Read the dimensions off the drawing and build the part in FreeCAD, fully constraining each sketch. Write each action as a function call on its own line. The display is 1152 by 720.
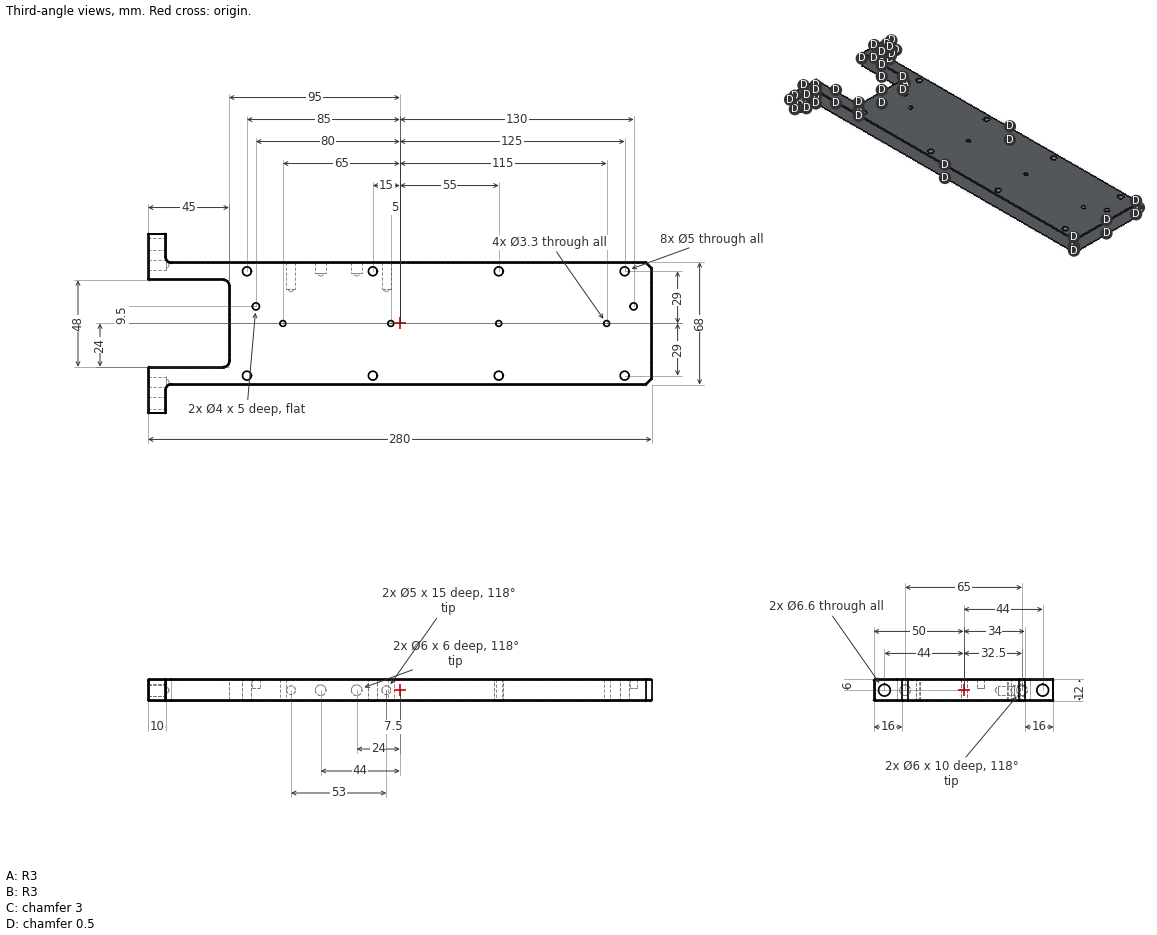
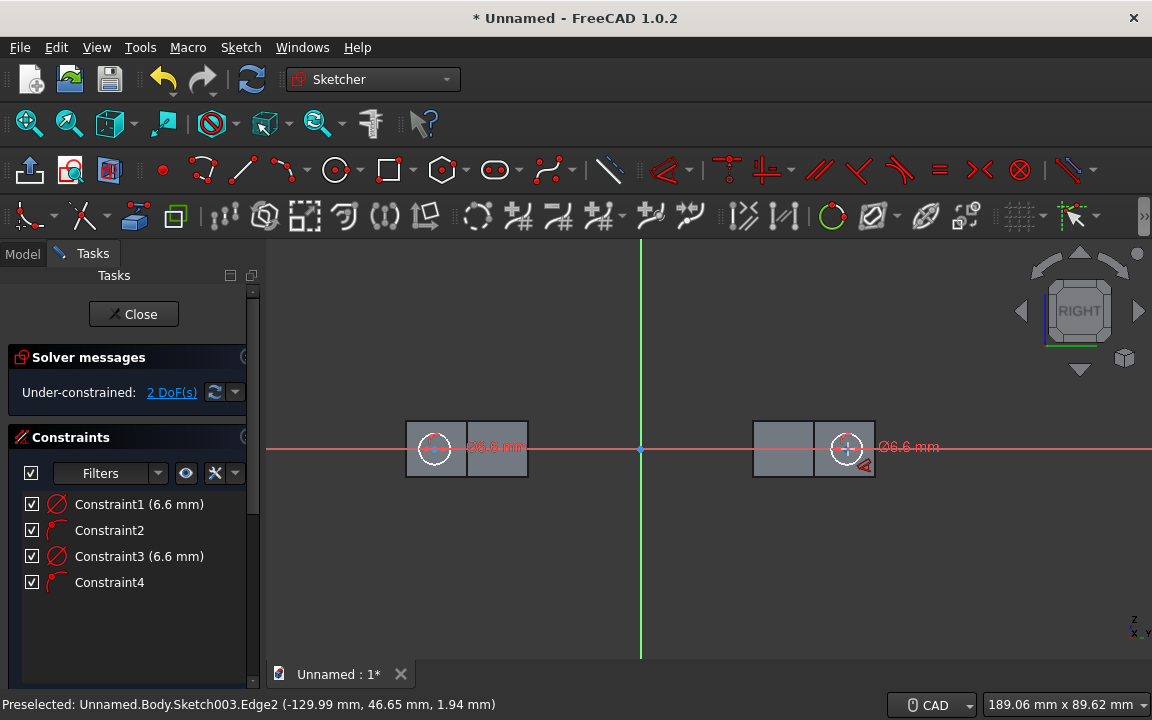
click(435, 449)
click(538, 483)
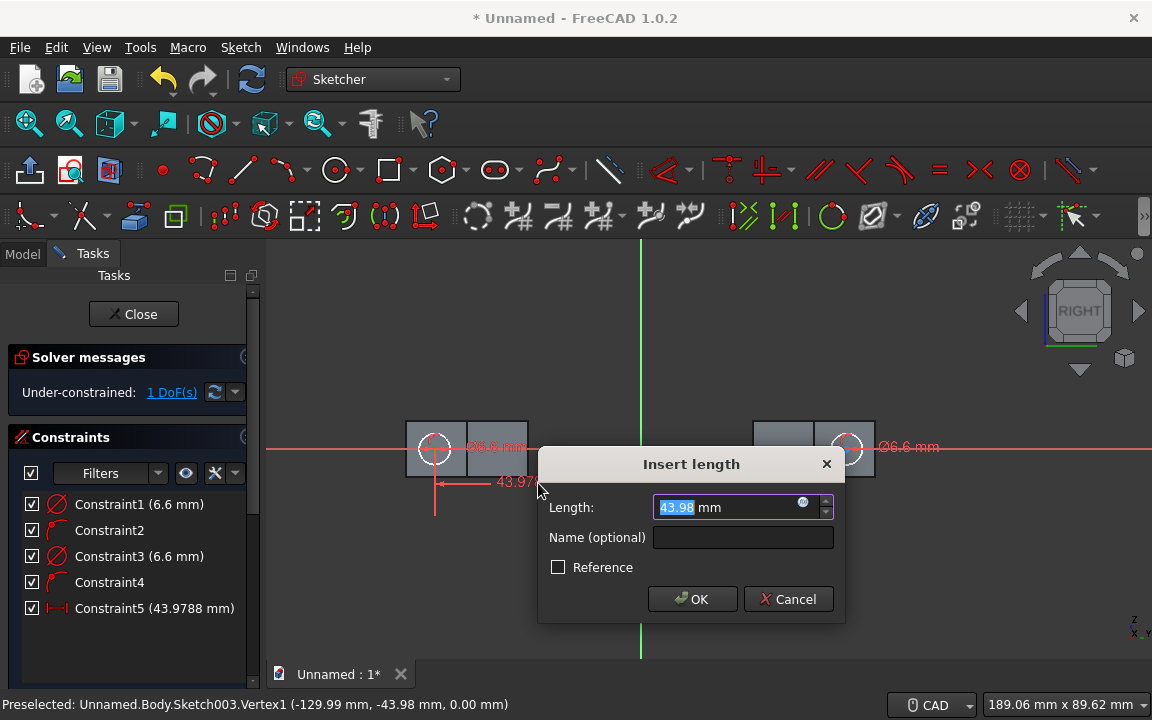
text(44)
key(Return)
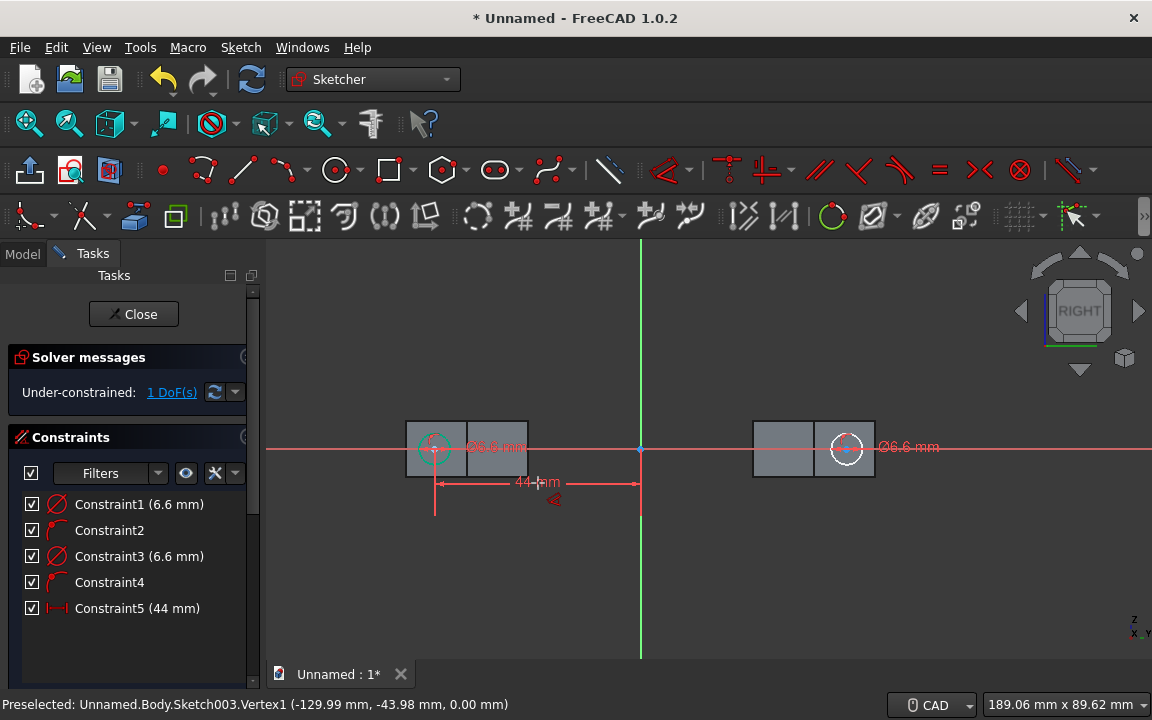
click(847, 449)
click(744, 483)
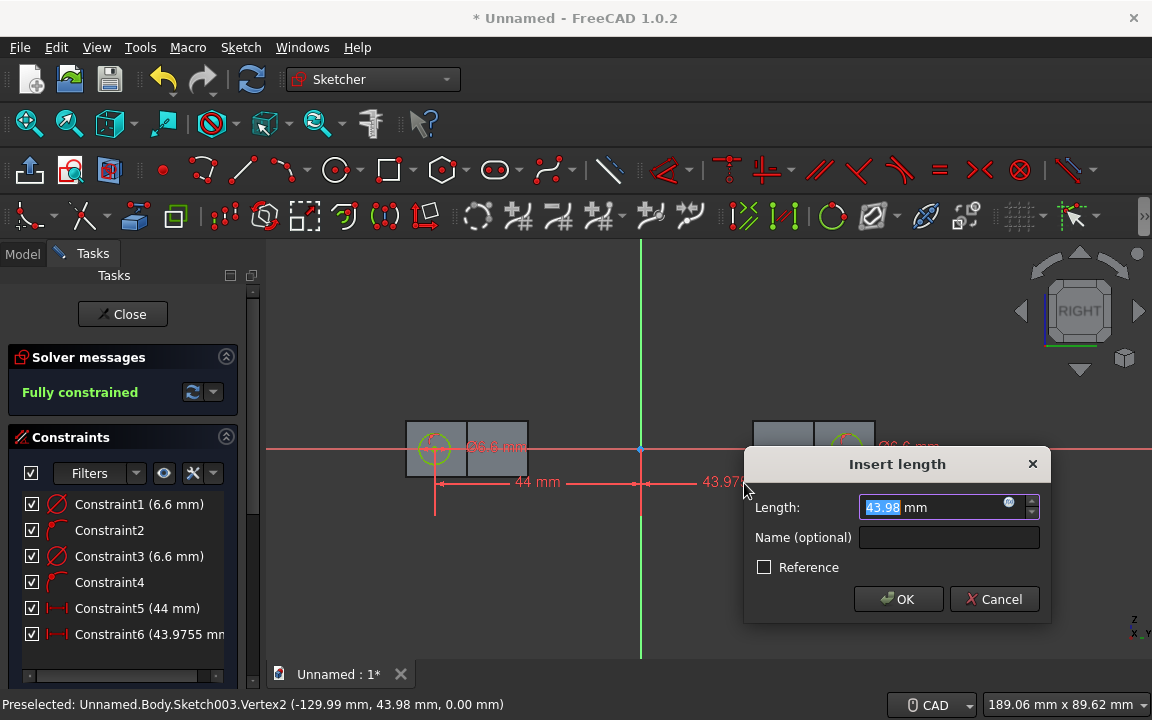
text(44)
key(Return)
key(Escape)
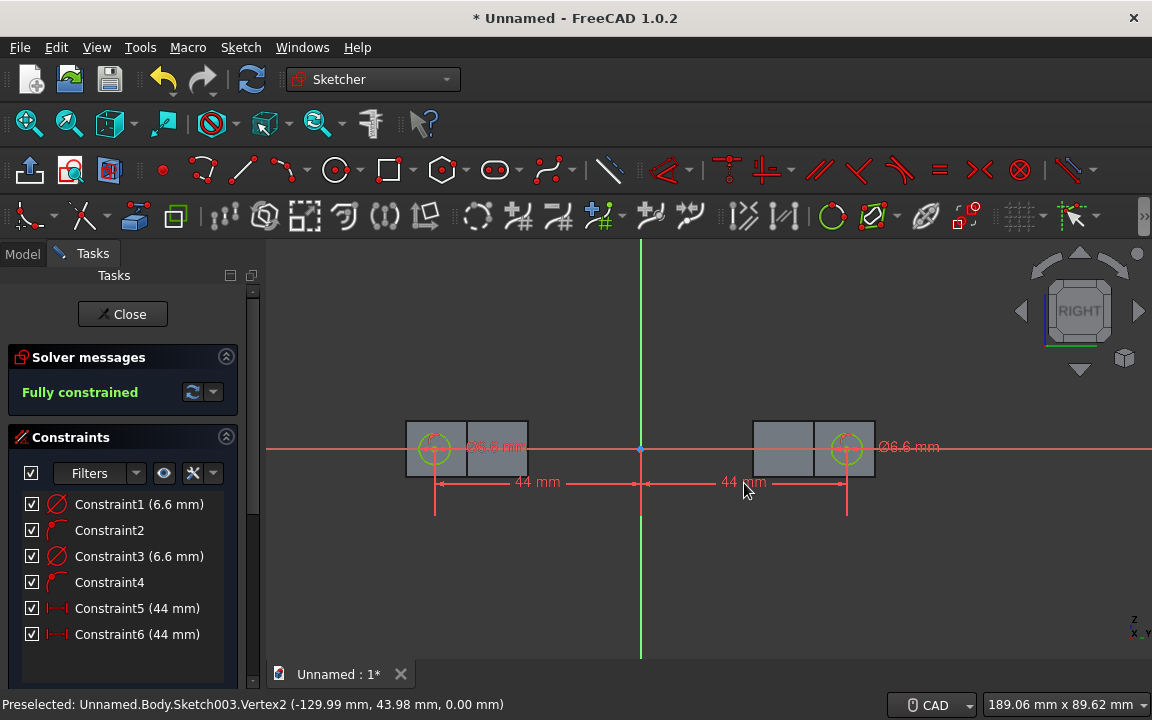
click(123, 314)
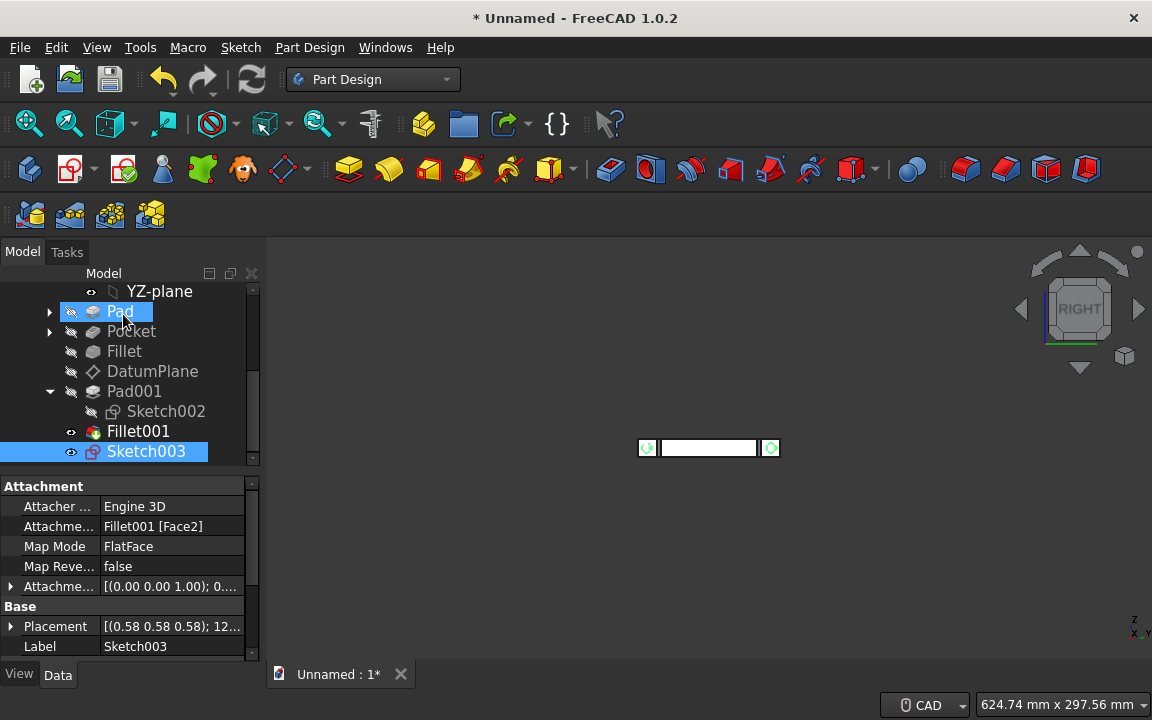
click(652, 170)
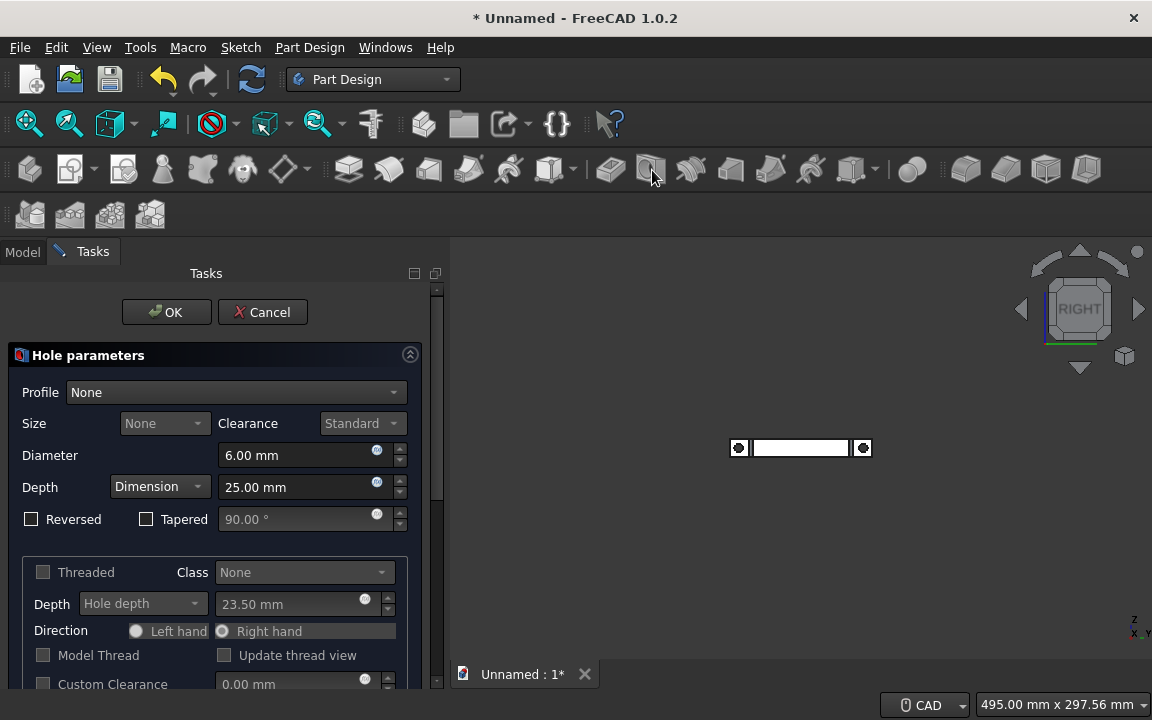
triple_click(305, 455)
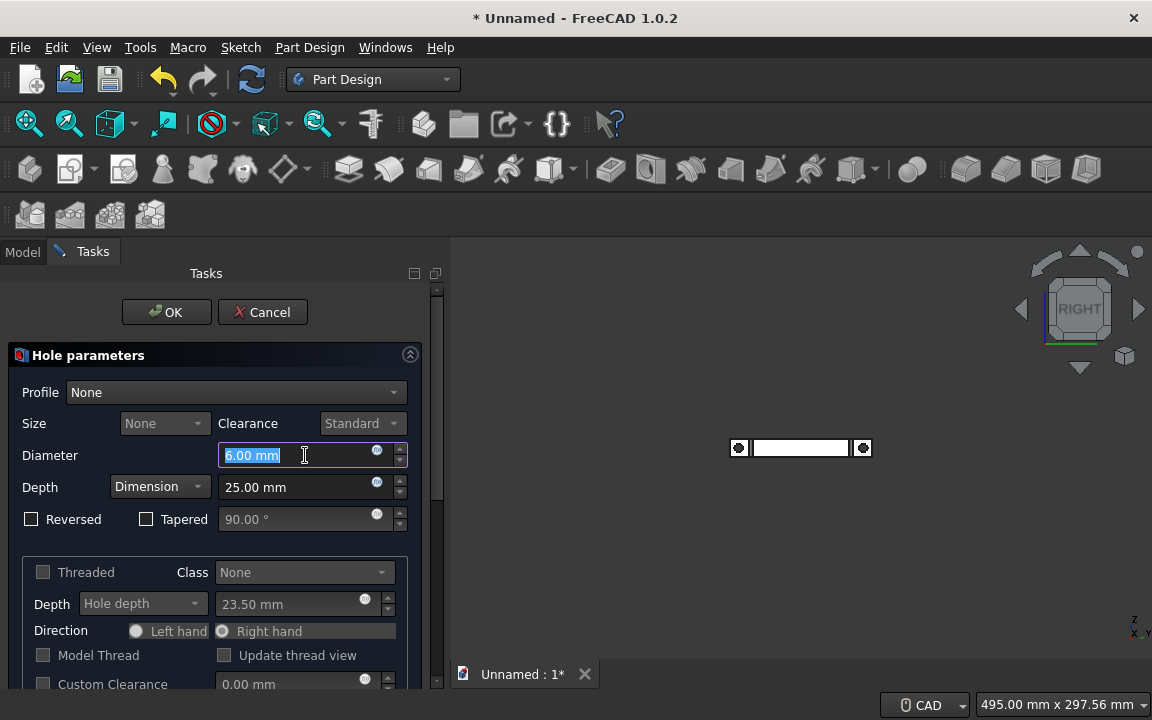
text(6.6)
key(Tab)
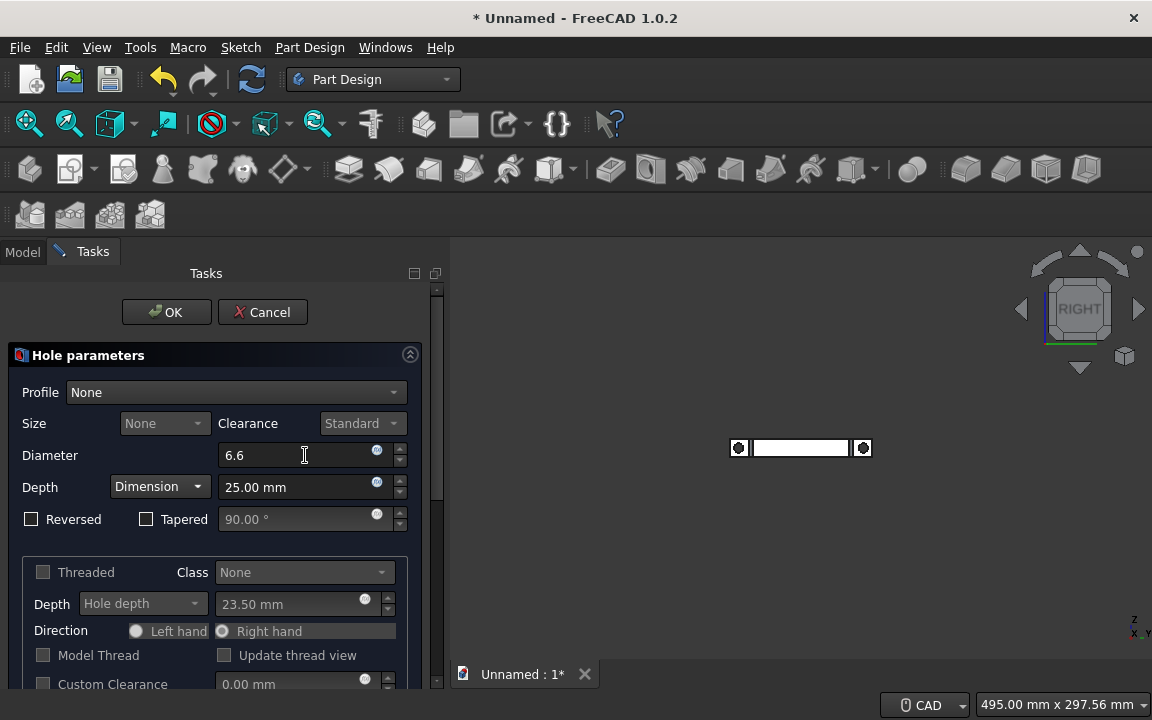
click(161, 486)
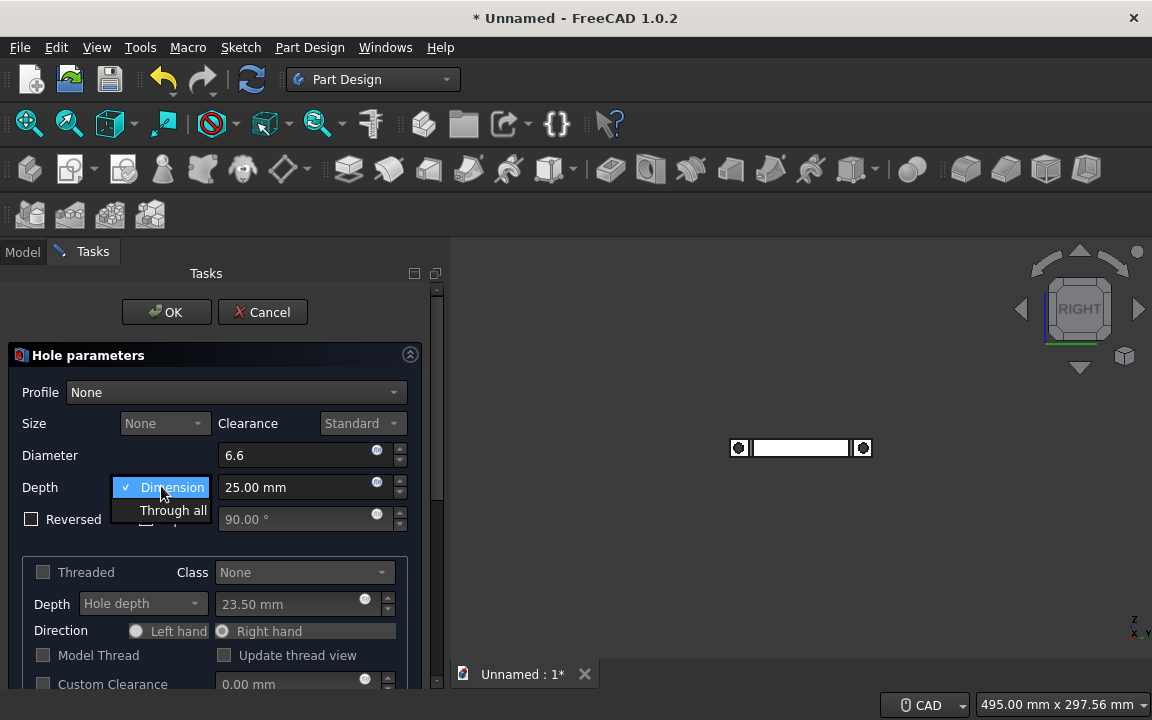
click(160, 510)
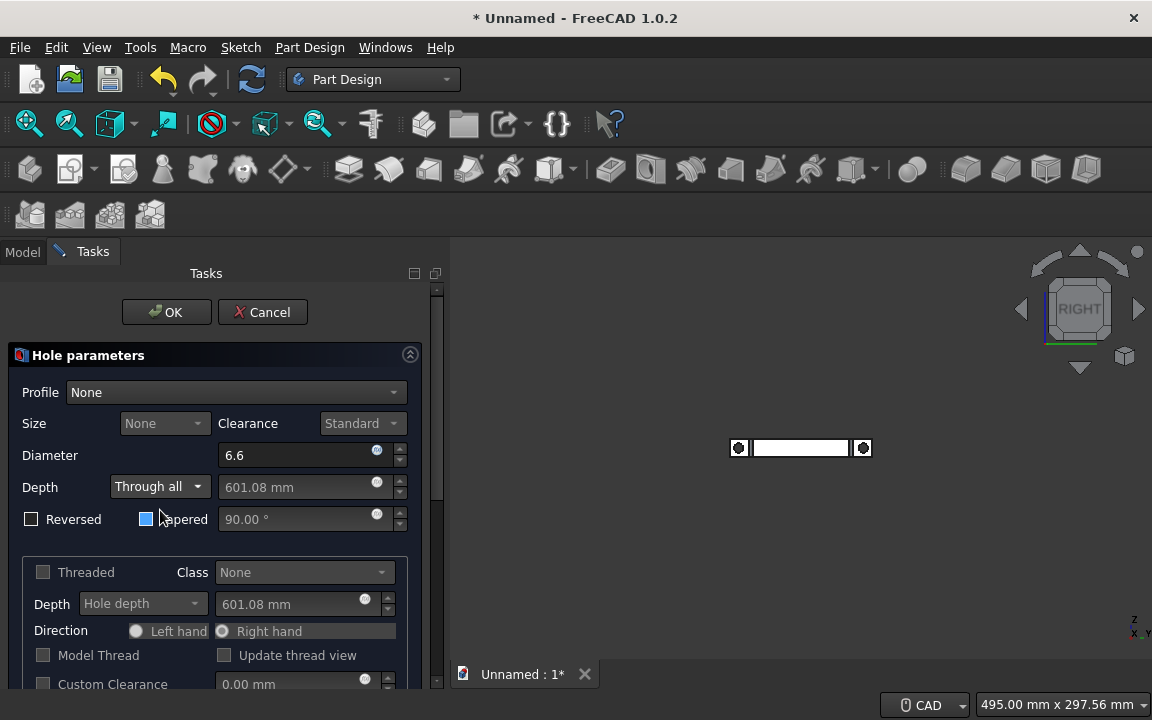
click(167, 312)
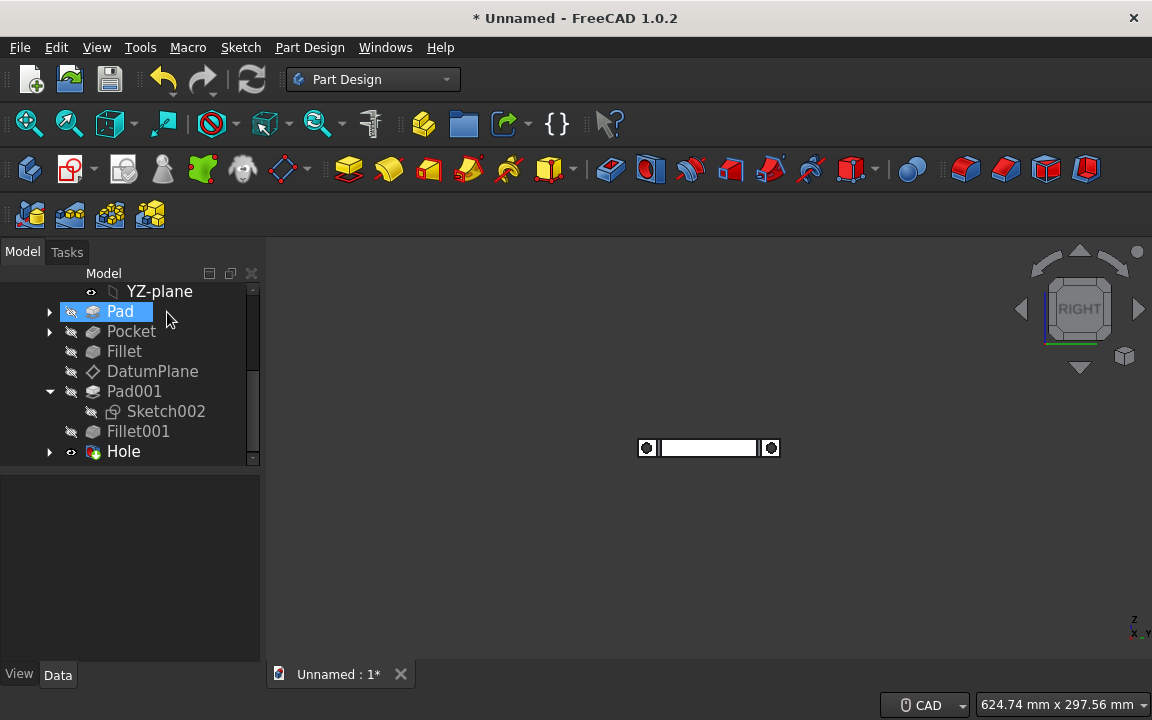
click(30, 124)